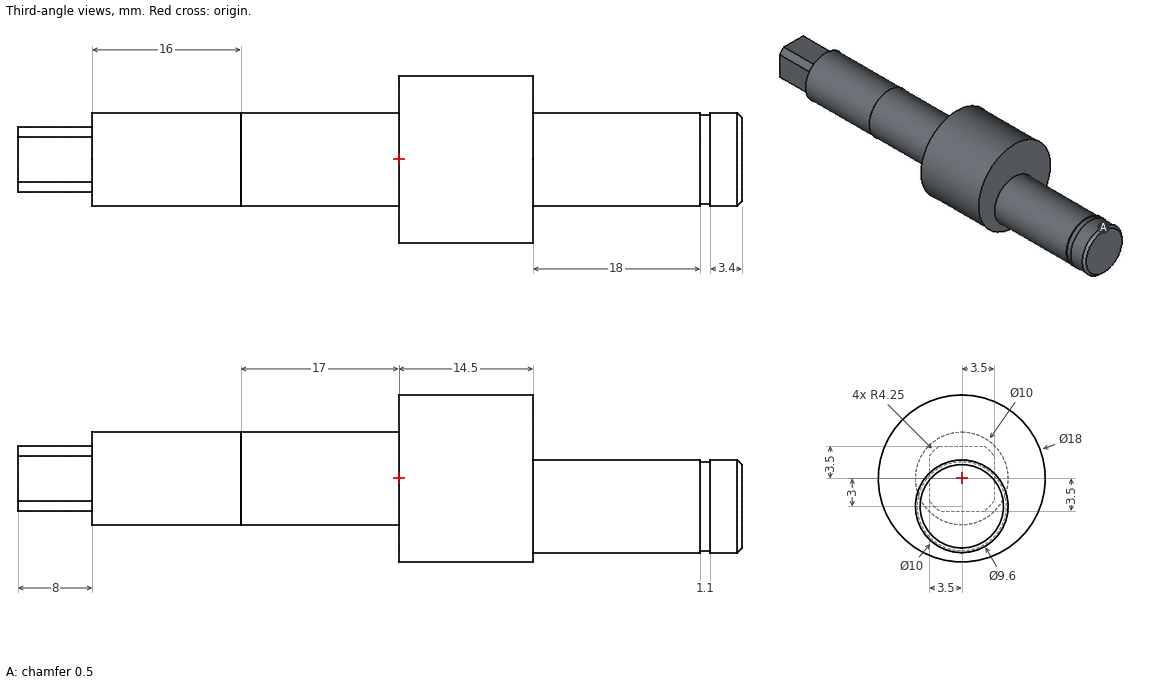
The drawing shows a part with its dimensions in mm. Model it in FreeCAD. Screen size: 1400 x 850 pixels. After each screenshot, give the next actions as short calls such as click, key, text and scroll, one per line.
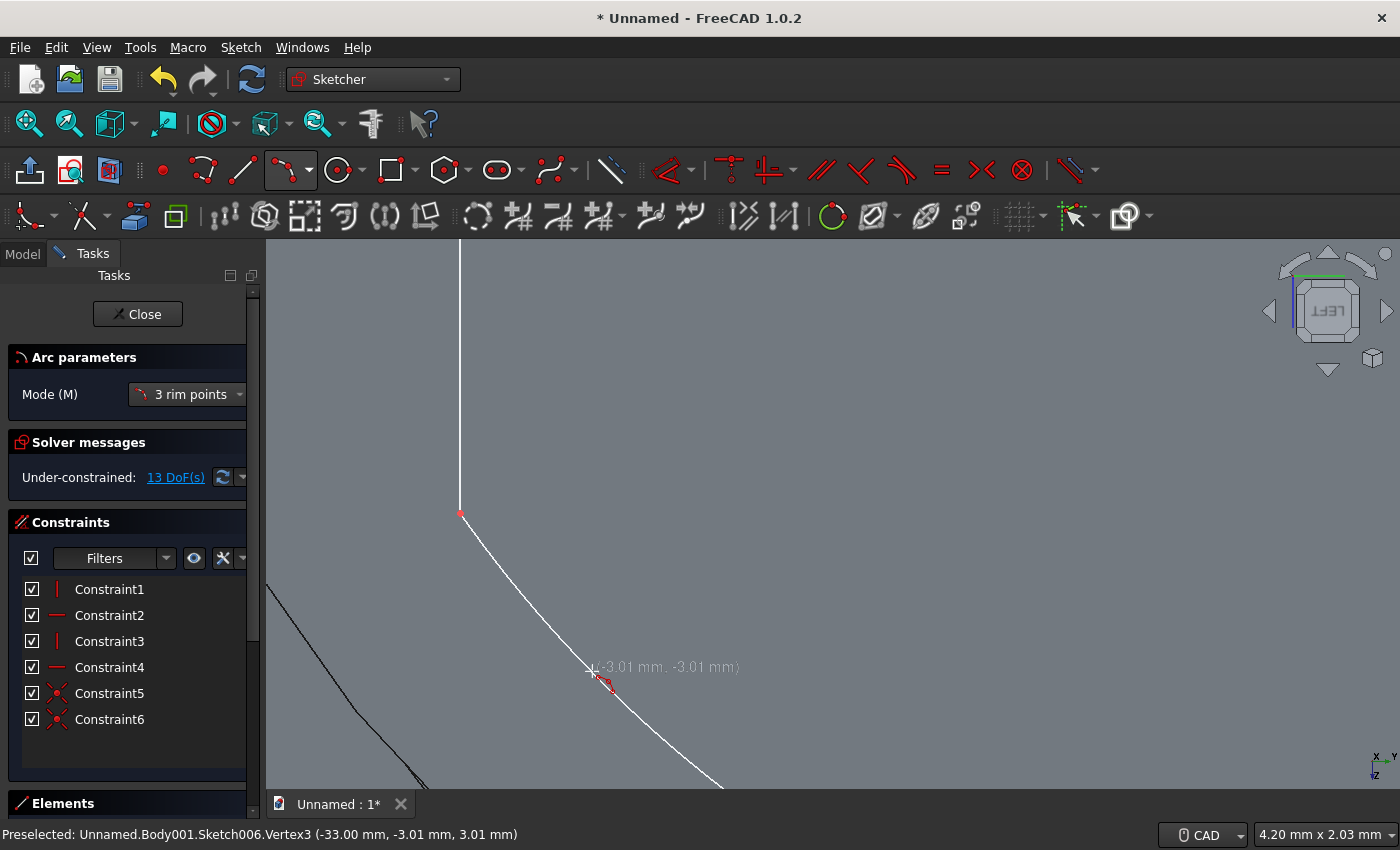
scroll(603, 680, down, 8)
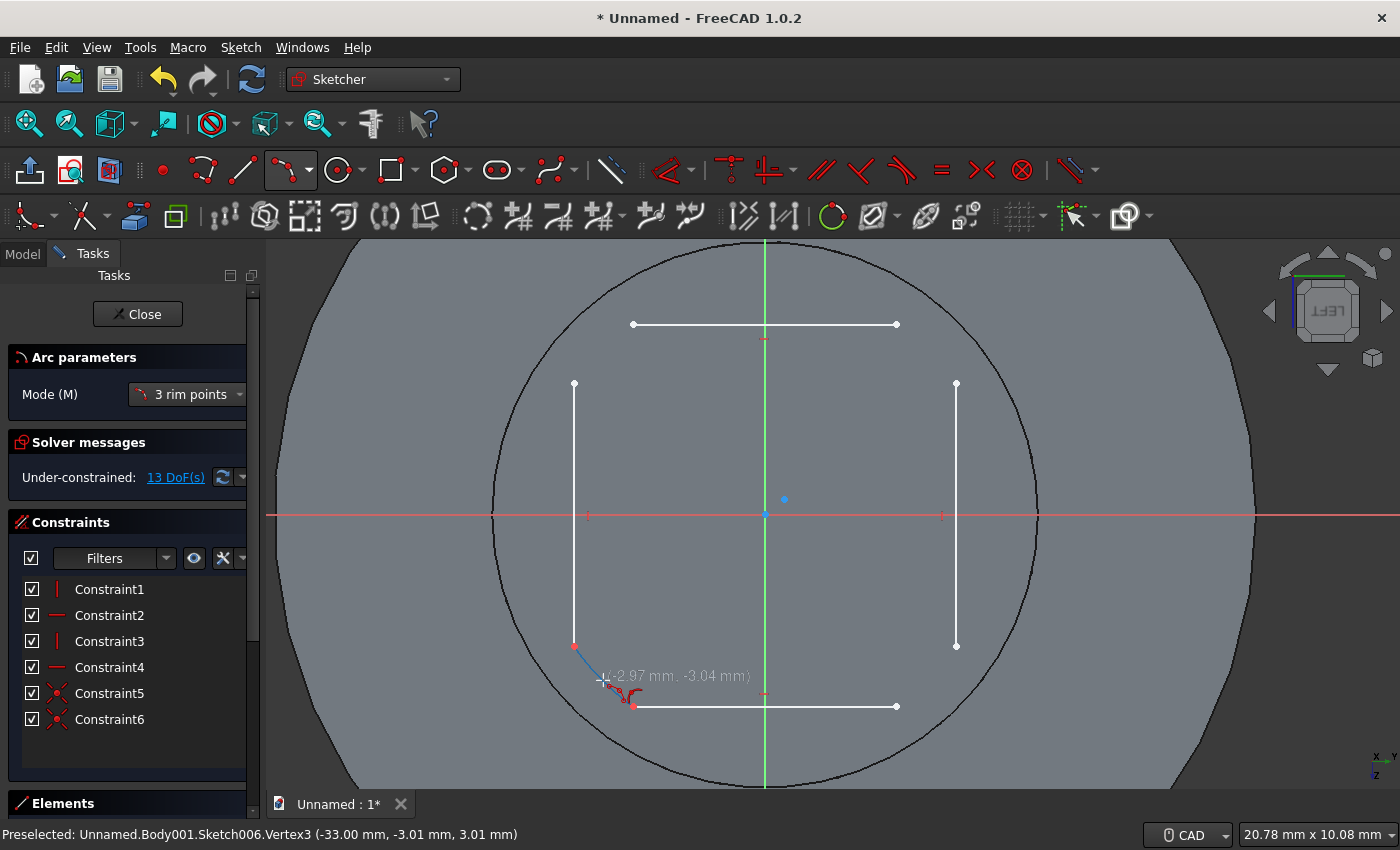
click(896, 707)
click(956, 647)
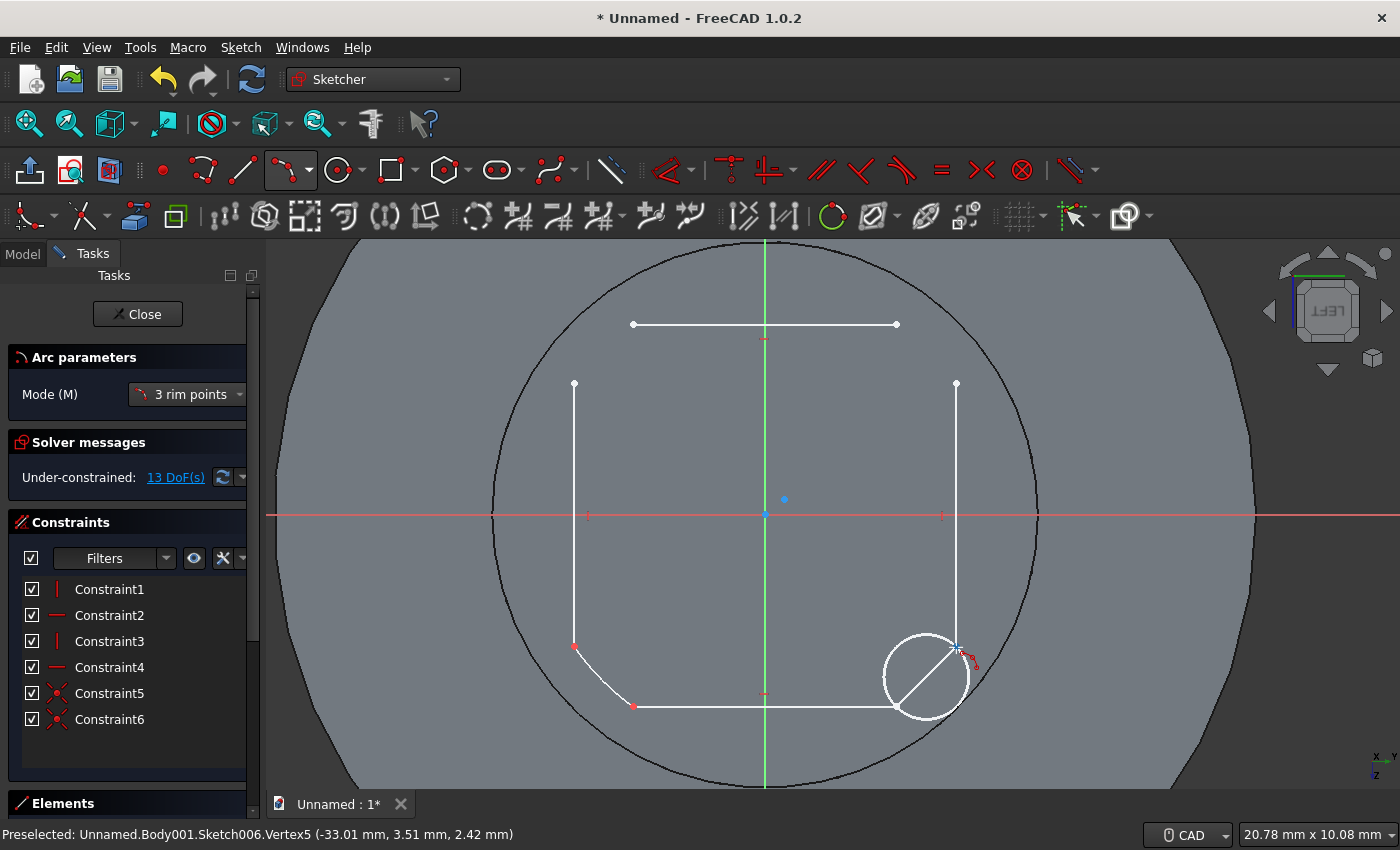
scroll(929, 679, up, 8)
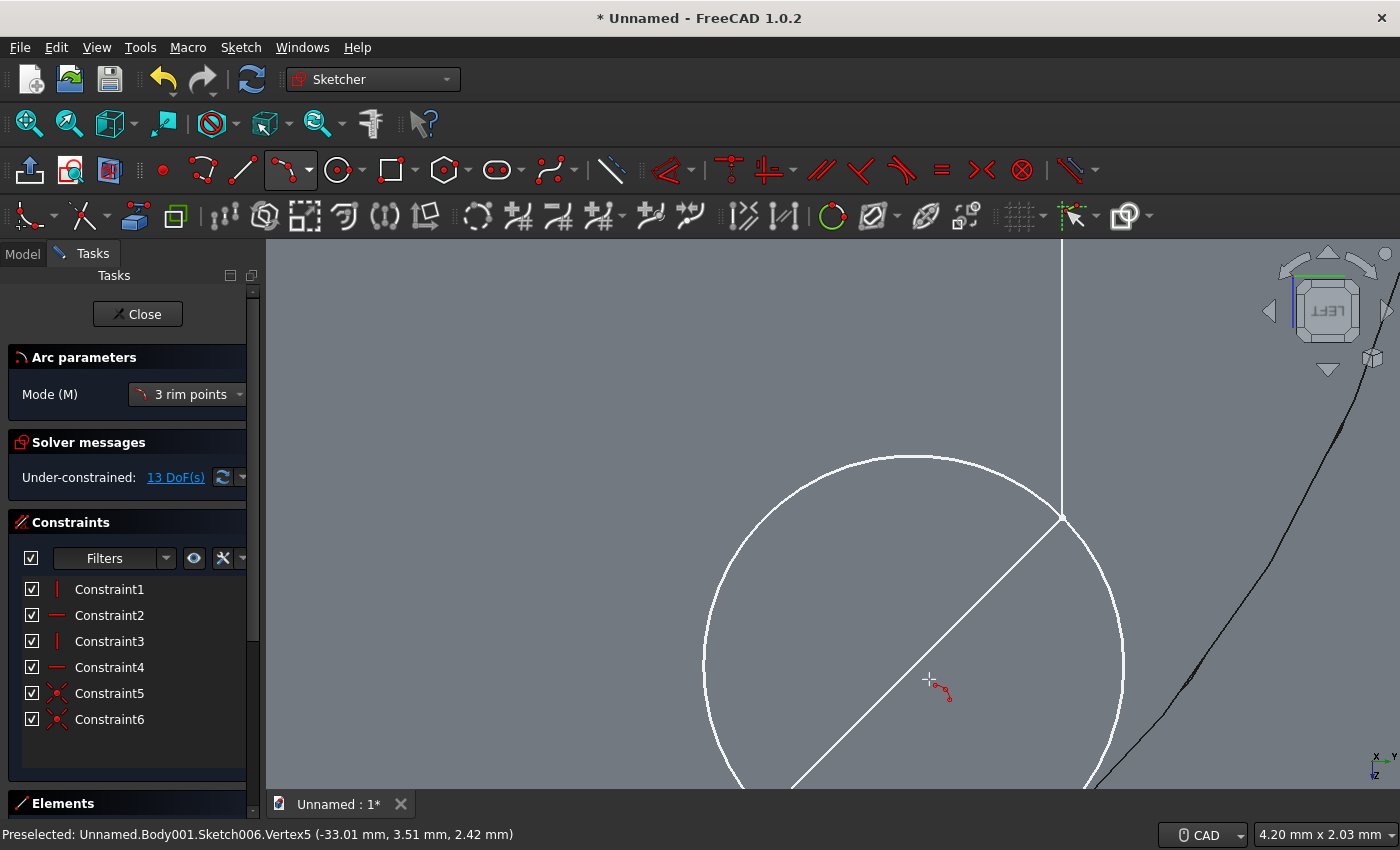
click(927, 675)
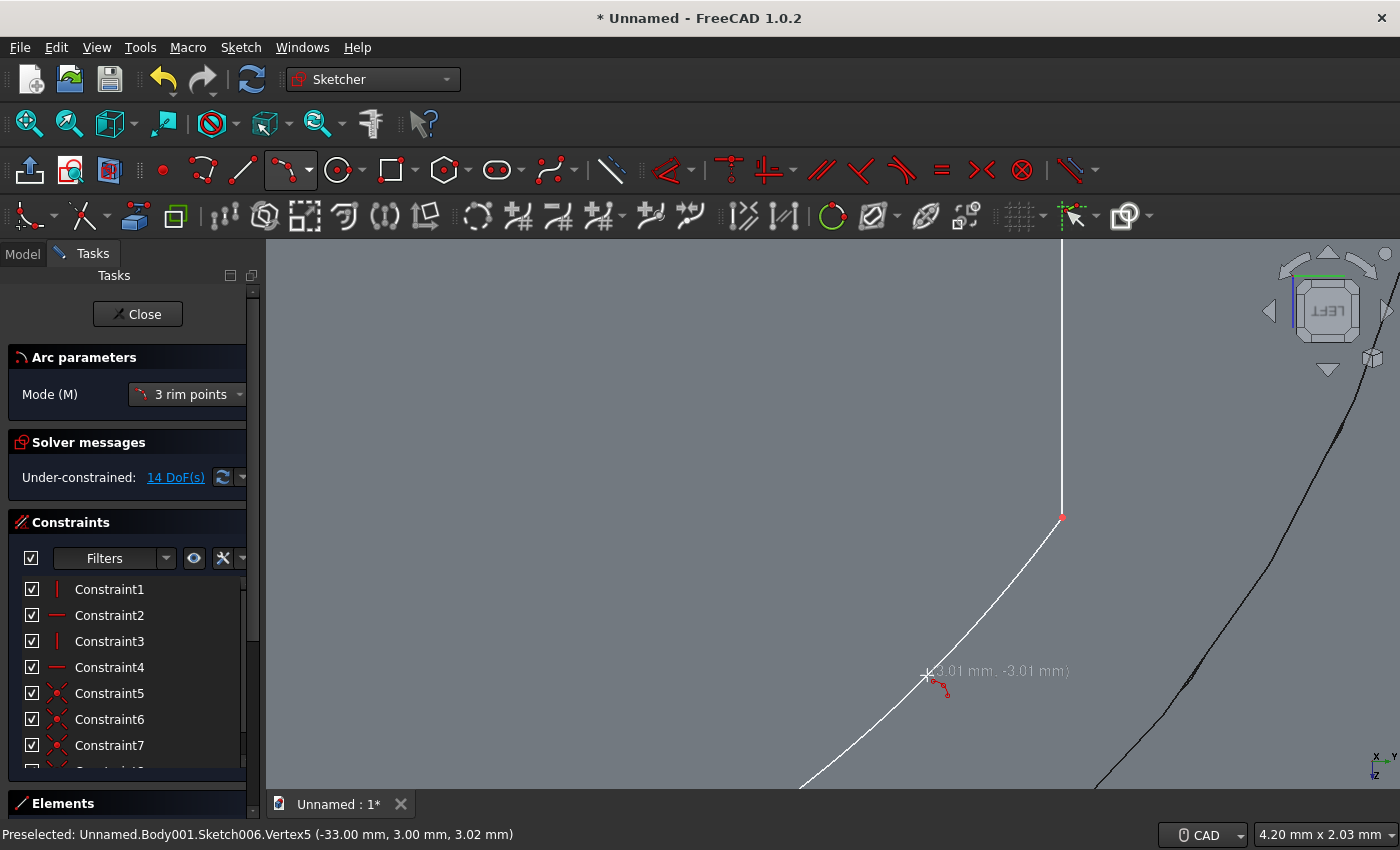
scroll(929, 679, down, 8)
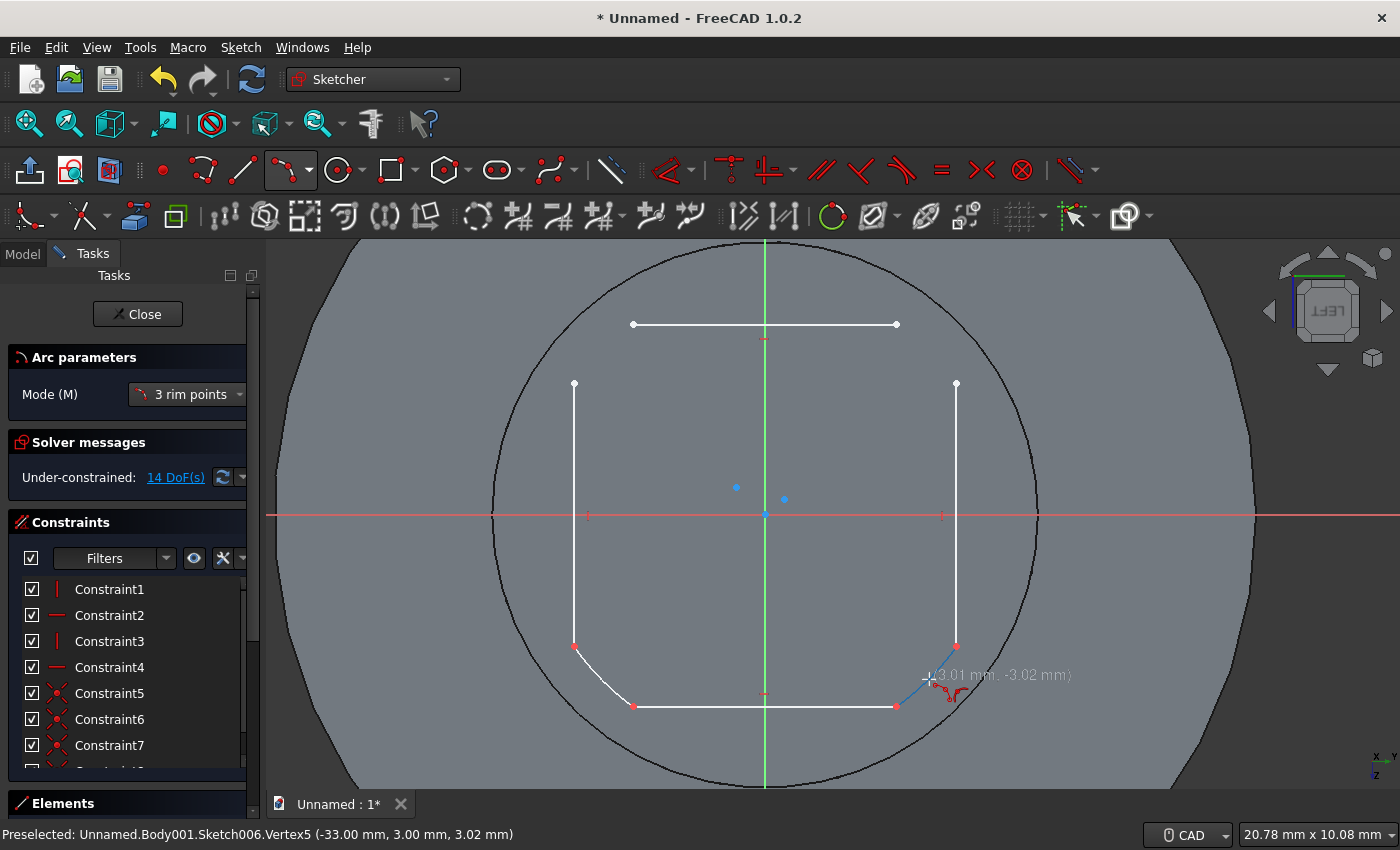
click(956, 384)
click(896, 325)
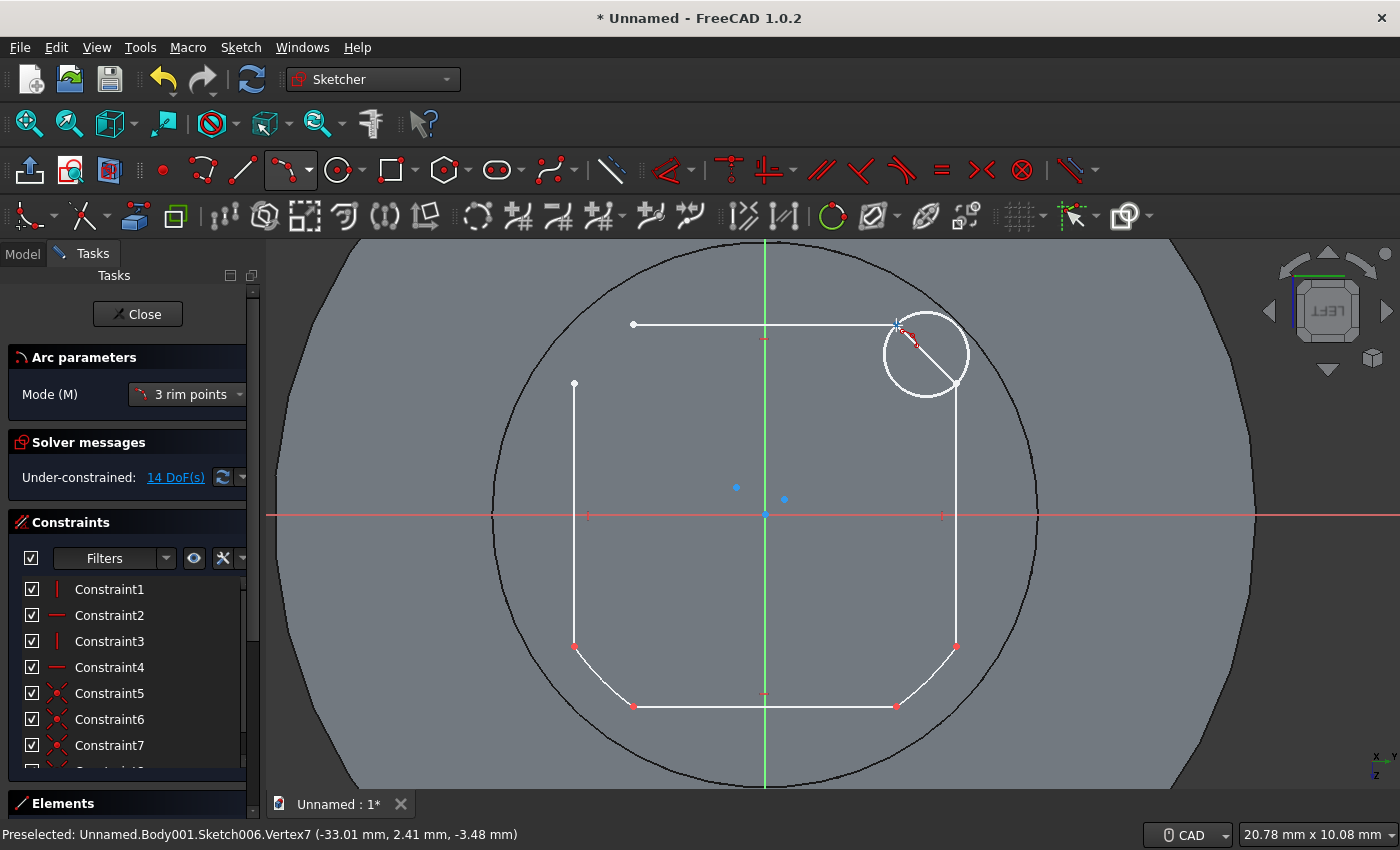
scroll(929, 351, up, 8)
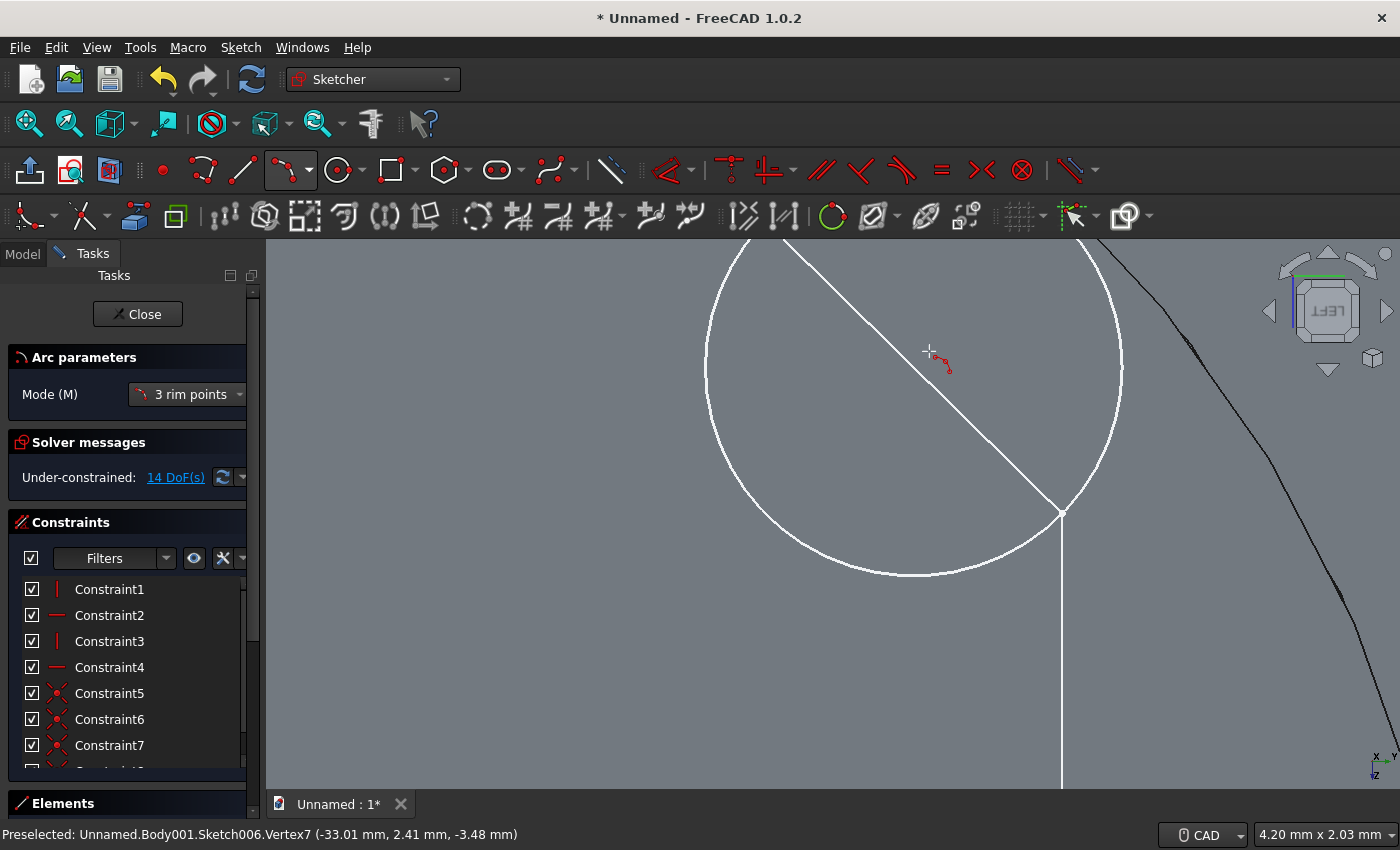
click(927, 349)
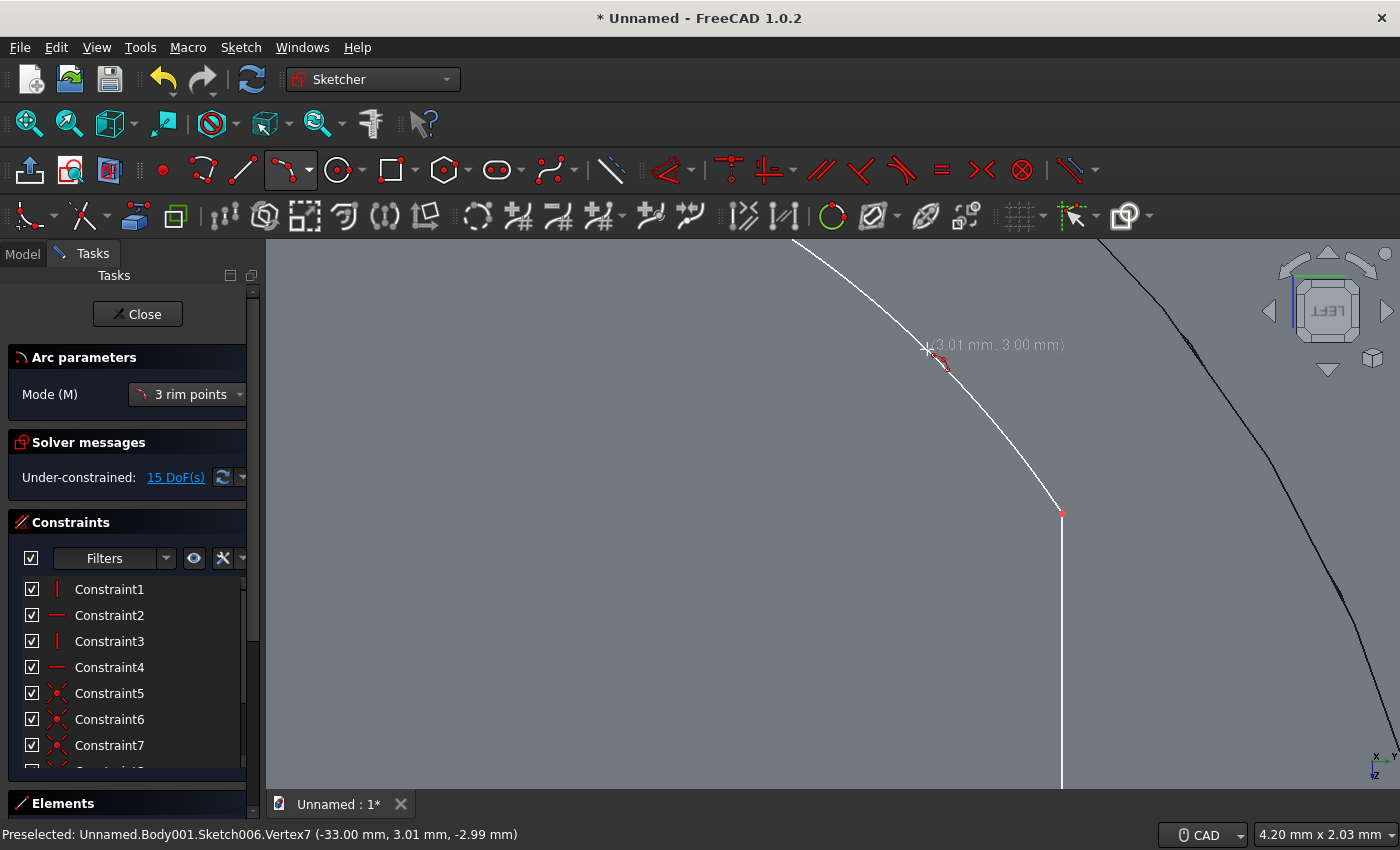
scroll(929, 350, down, 8)